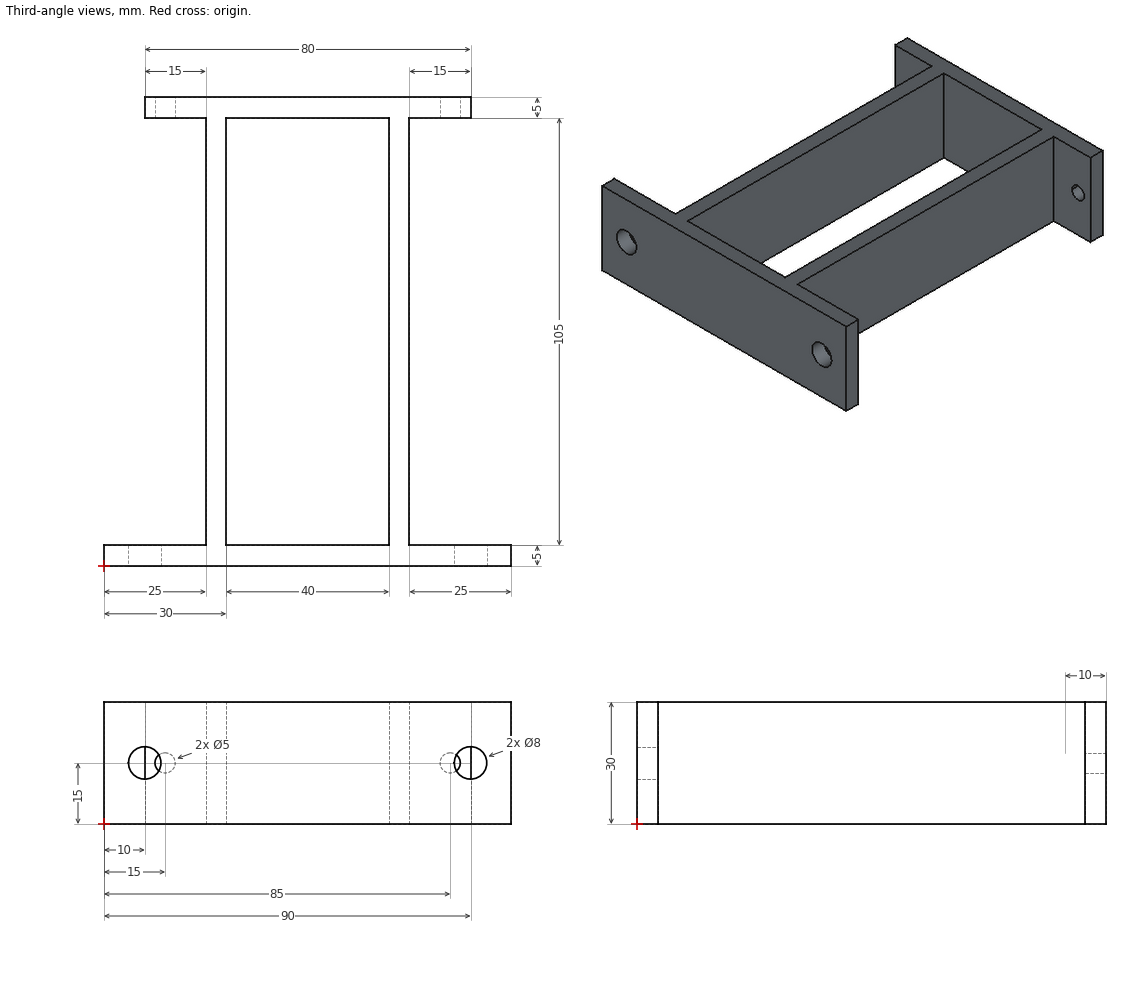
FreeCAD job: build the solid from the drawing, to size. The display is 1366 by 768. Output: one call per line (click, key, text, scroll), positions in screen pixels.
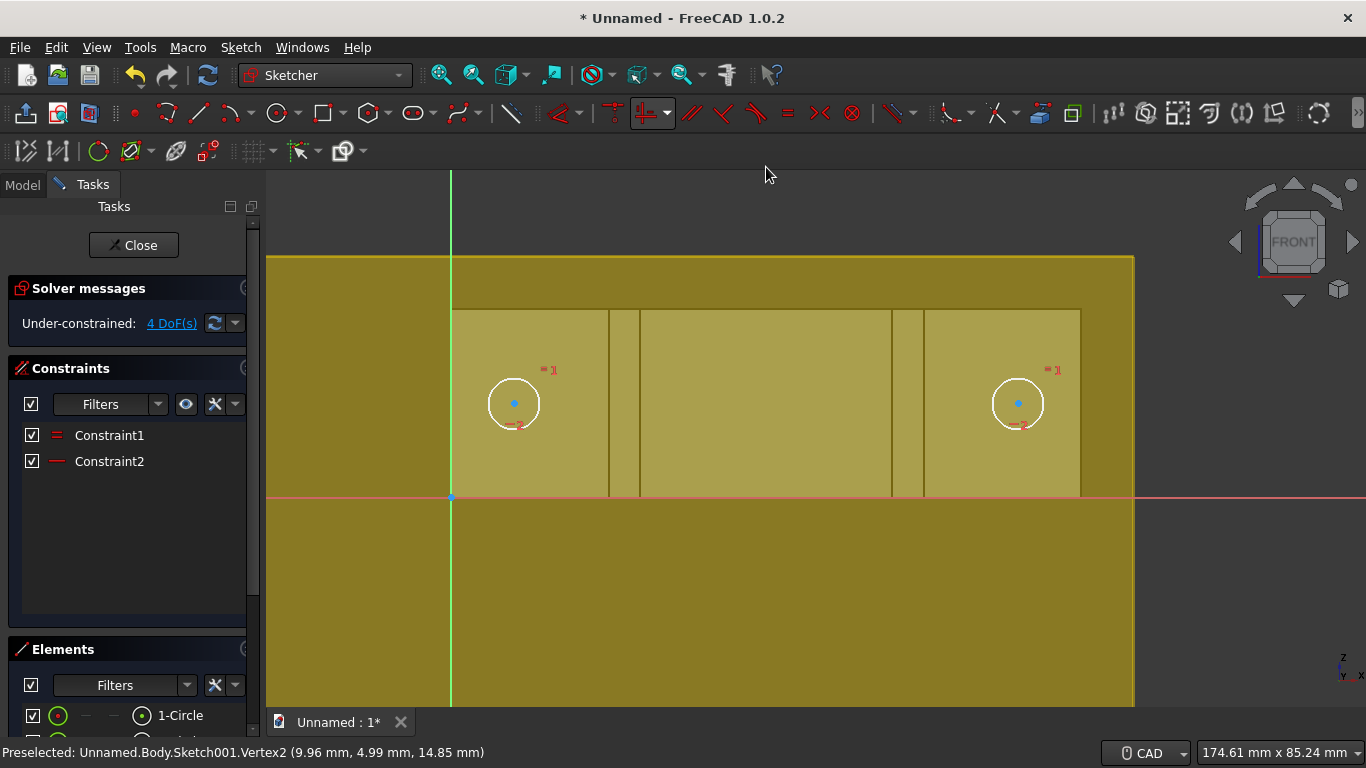
click(558, 114)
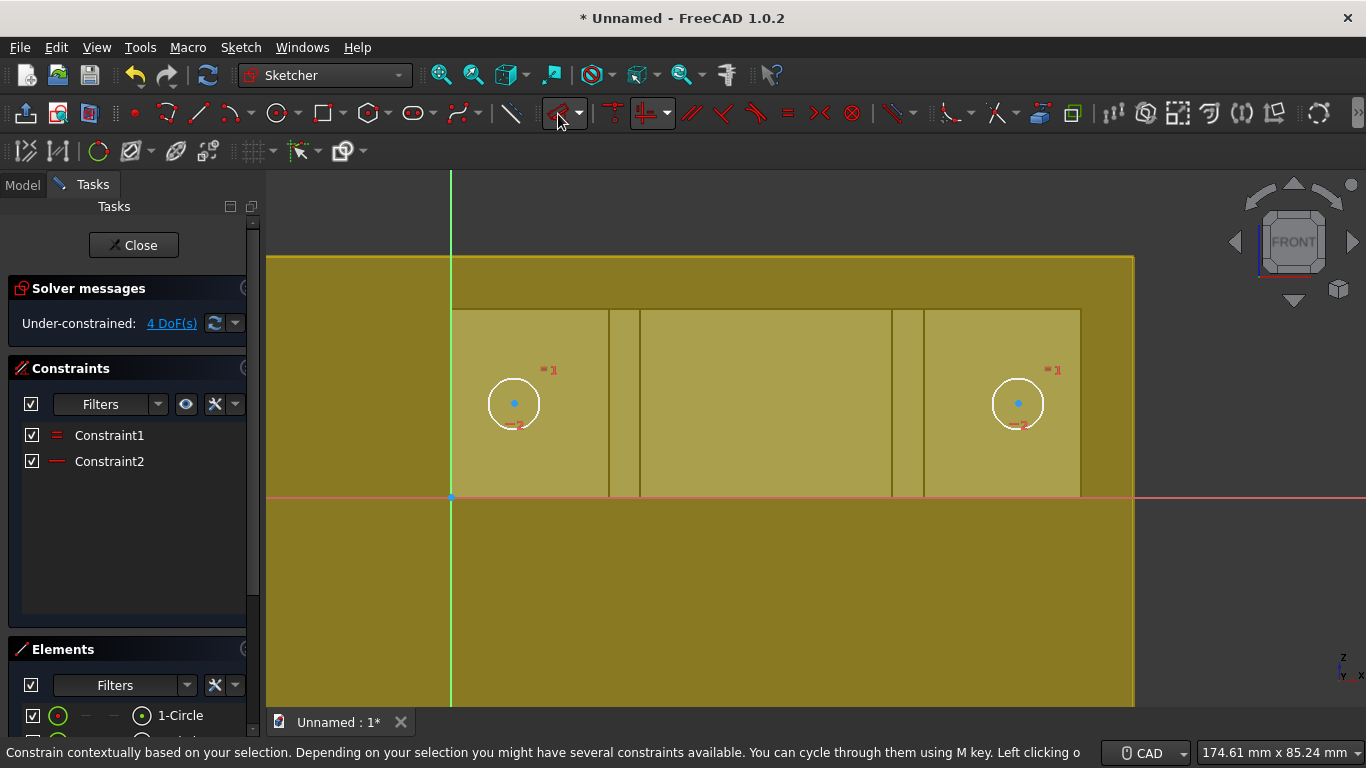
click(1036, 386)
click(1059, 363)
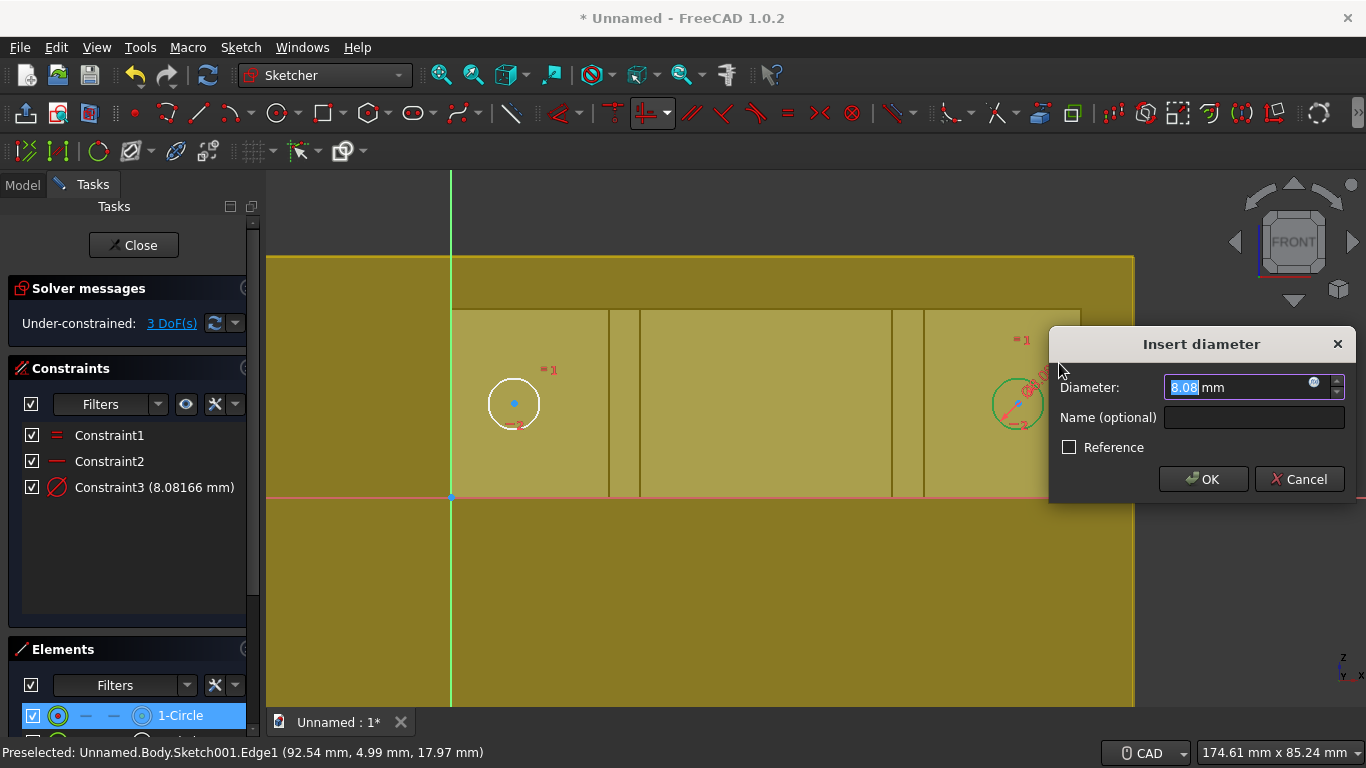
text(8)
key(Return)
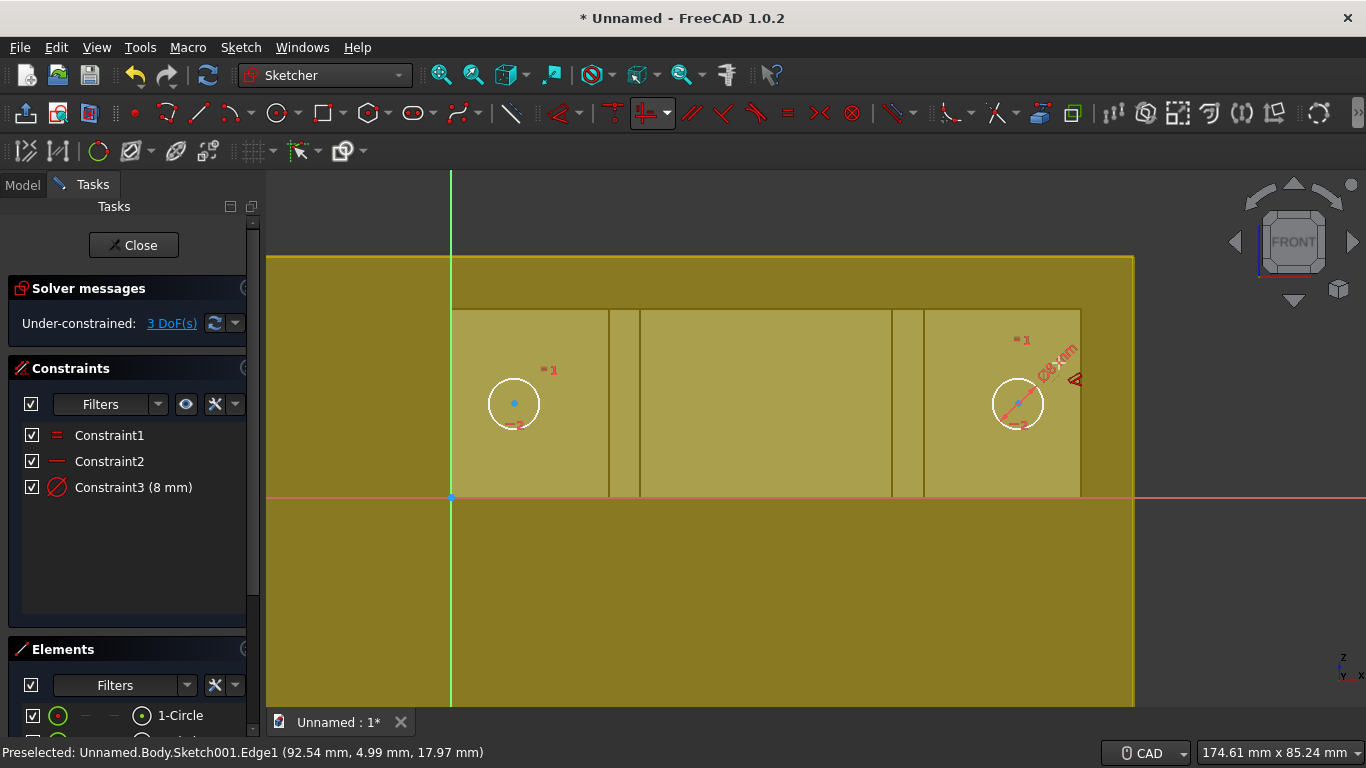
click(1018, 404)
click(735, 532)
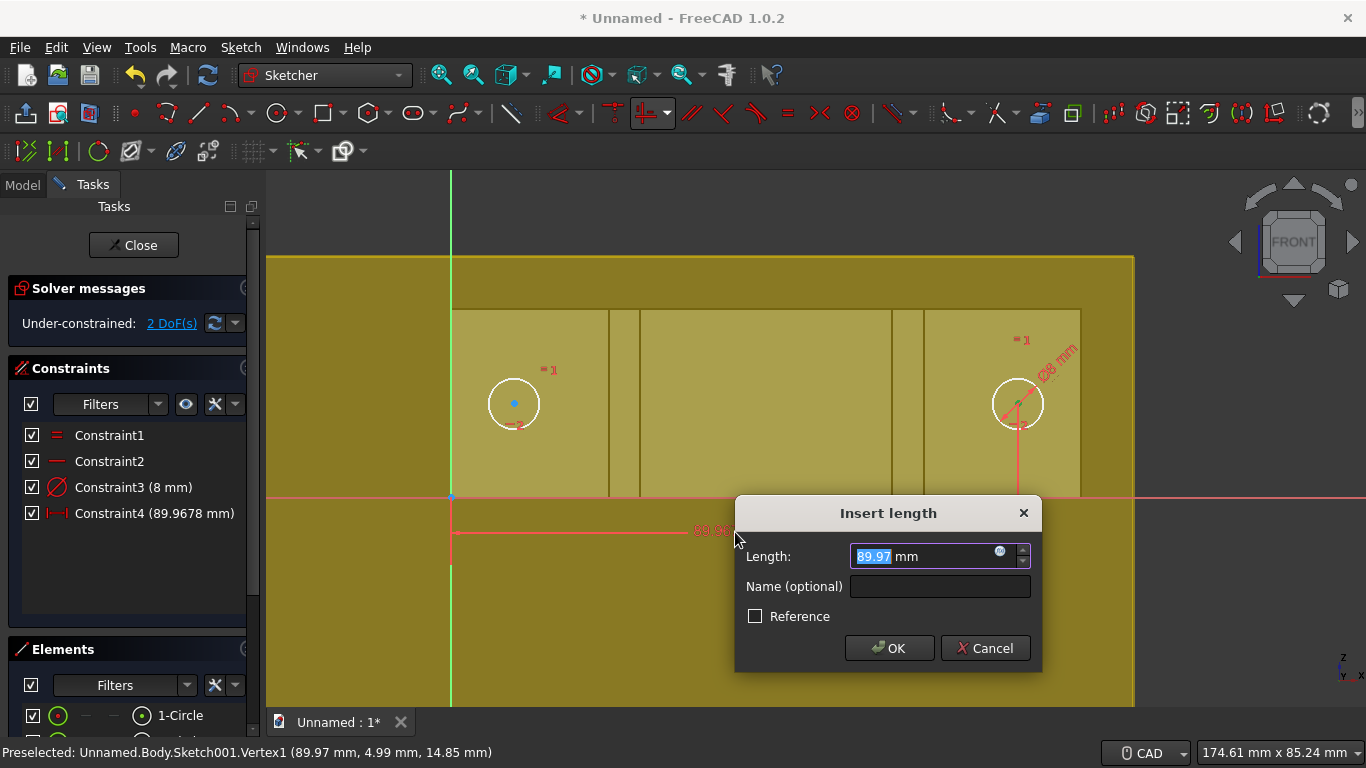
text(90)
key(Return)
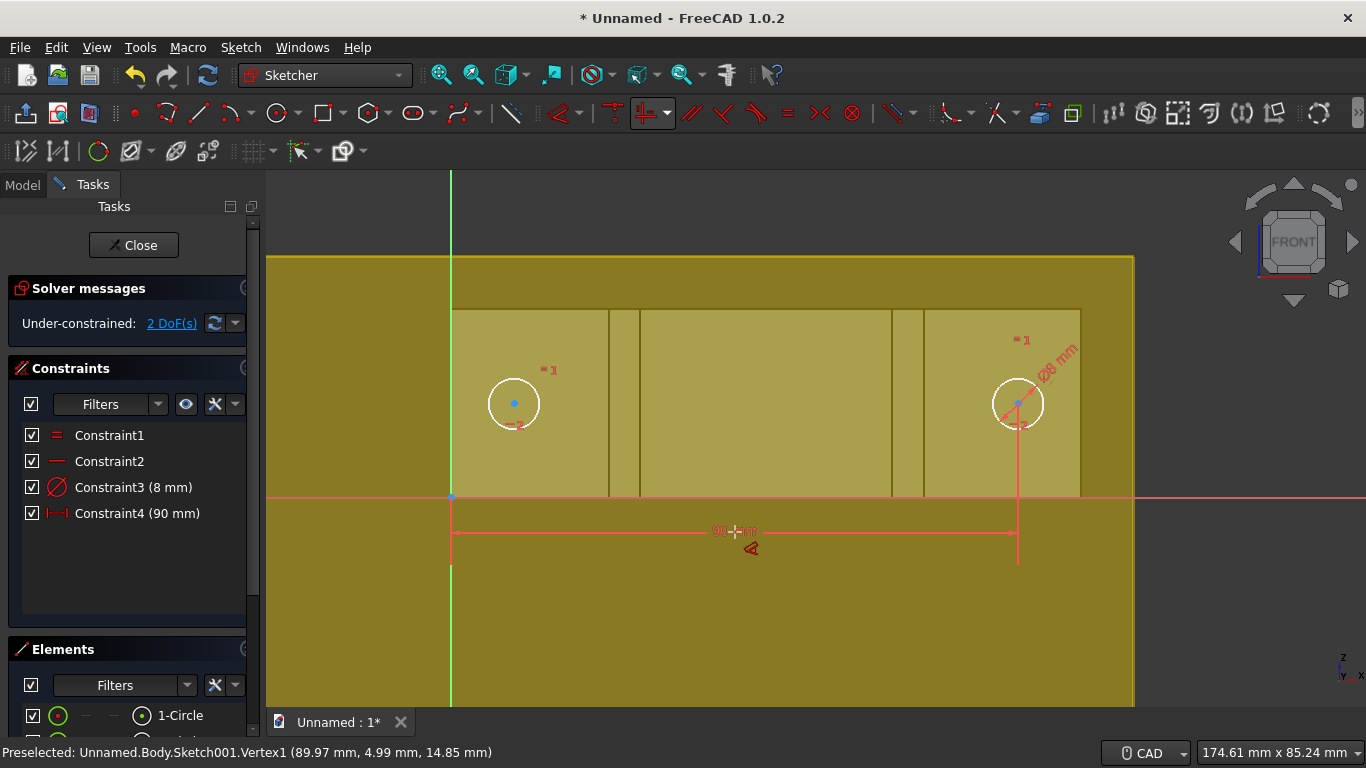
click(1018, 404)
click(417, 451)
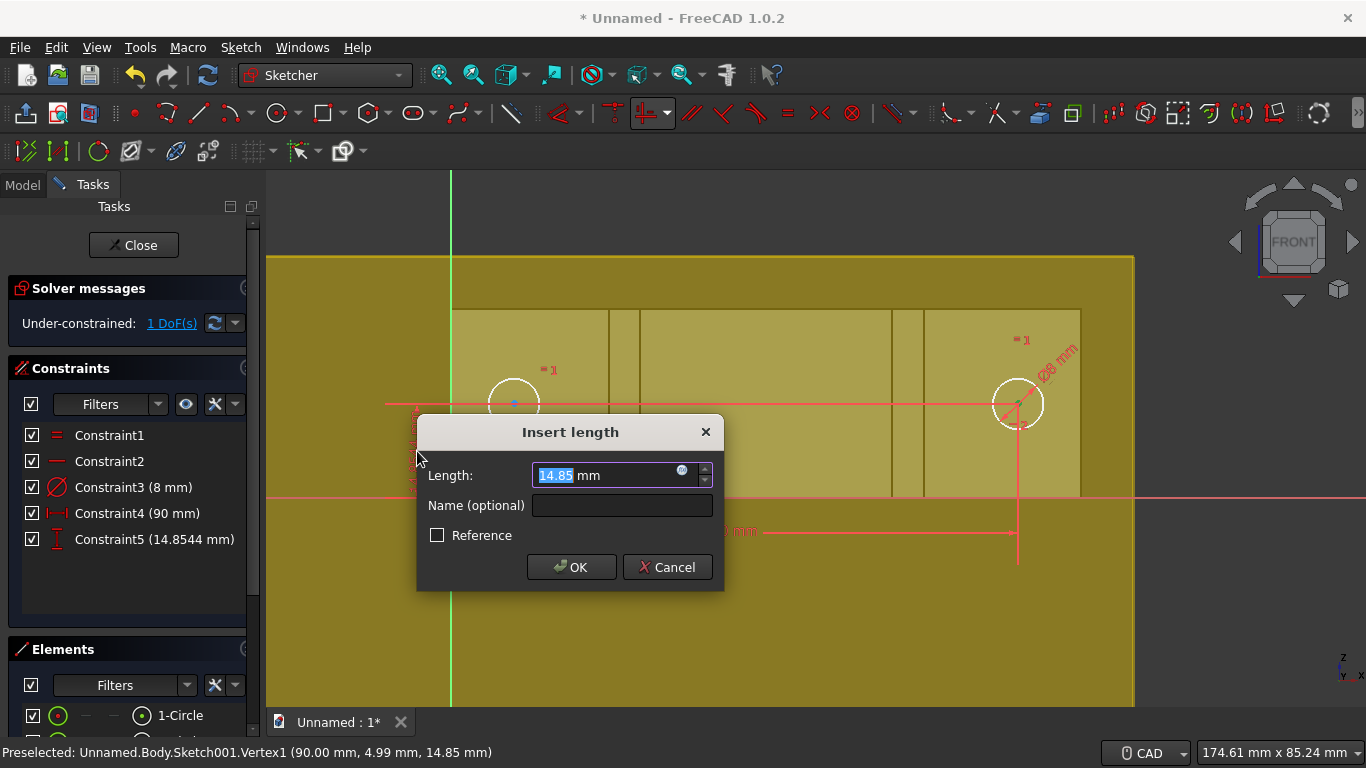
text(15)
key(Return)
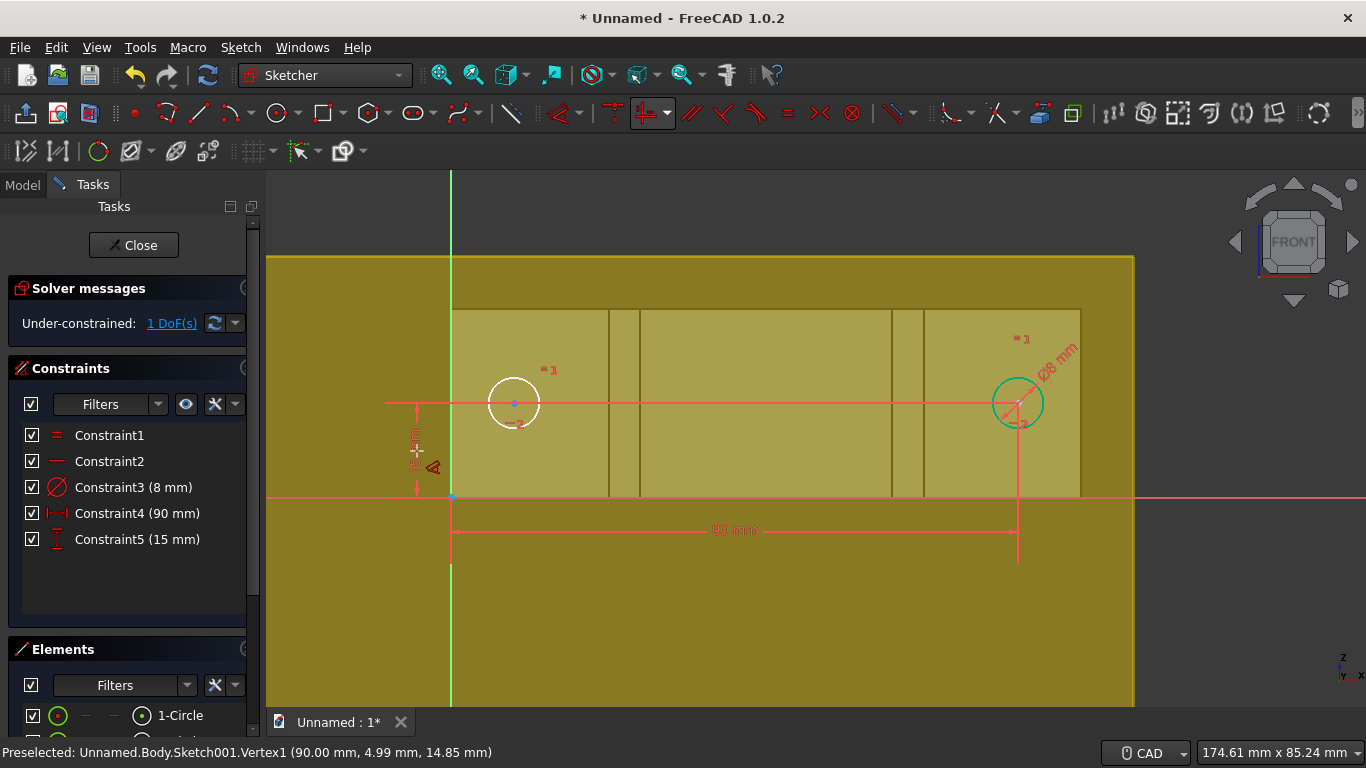
click(514, 403)
click(483, 532)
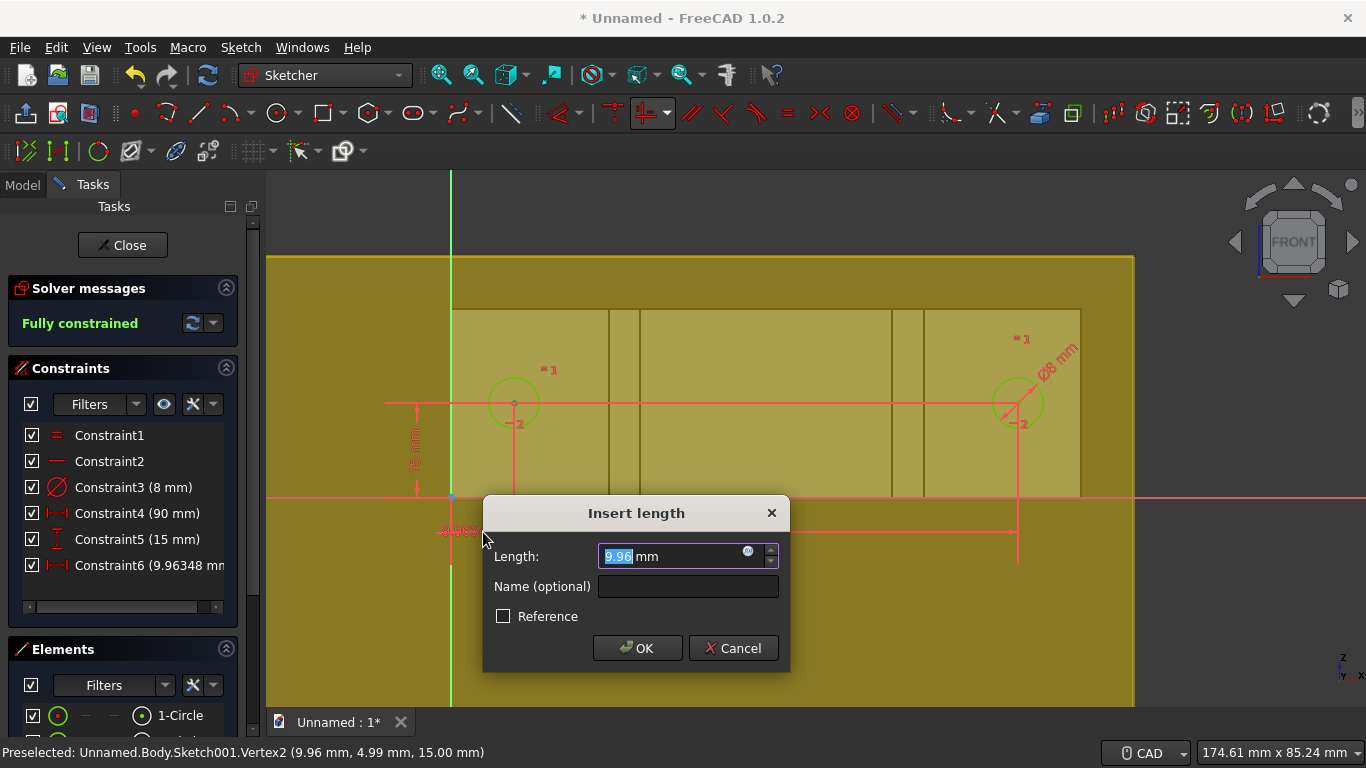
text(10)
key(Return)
key(Escape)